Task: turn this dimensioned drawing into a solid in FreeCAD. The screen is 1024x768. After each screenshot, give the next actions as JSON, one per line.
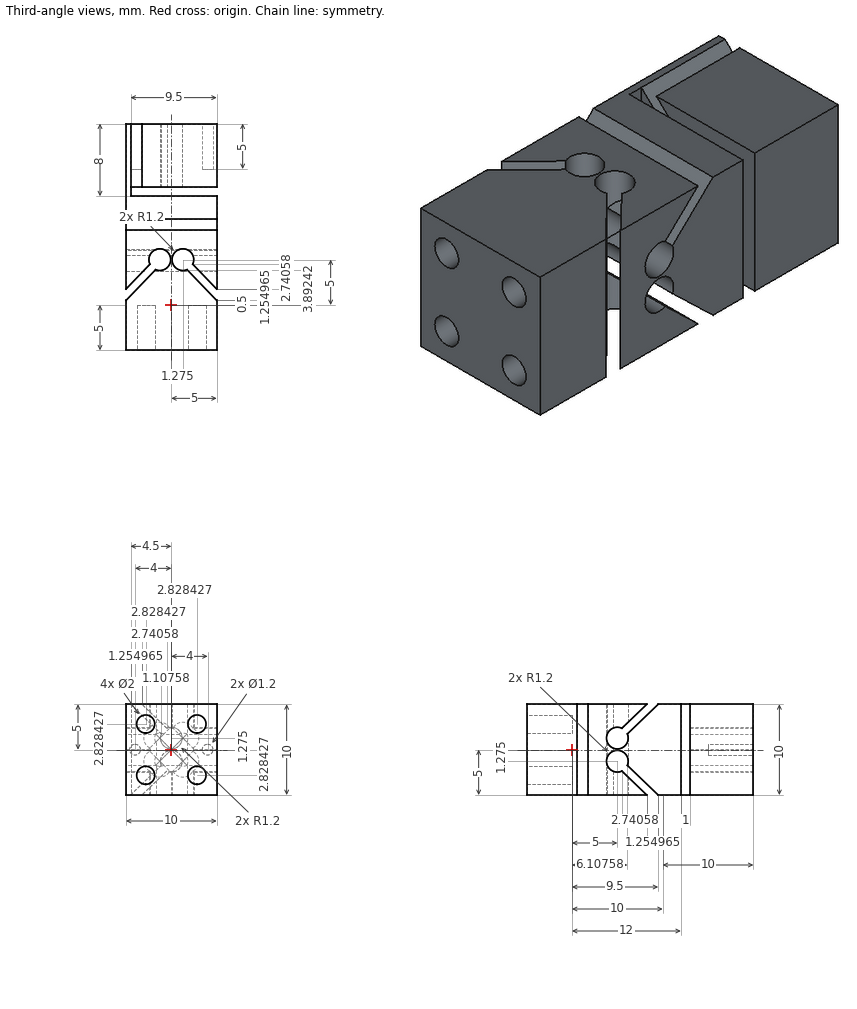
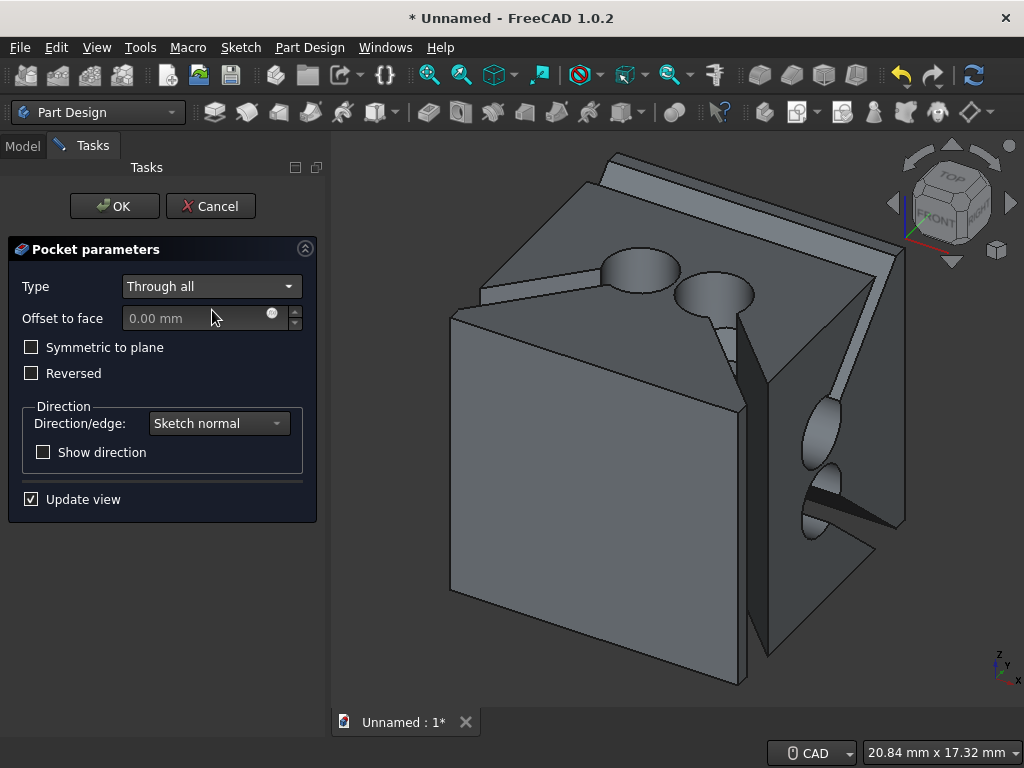
{"action": "left_click", "coordinate": [115, 206]}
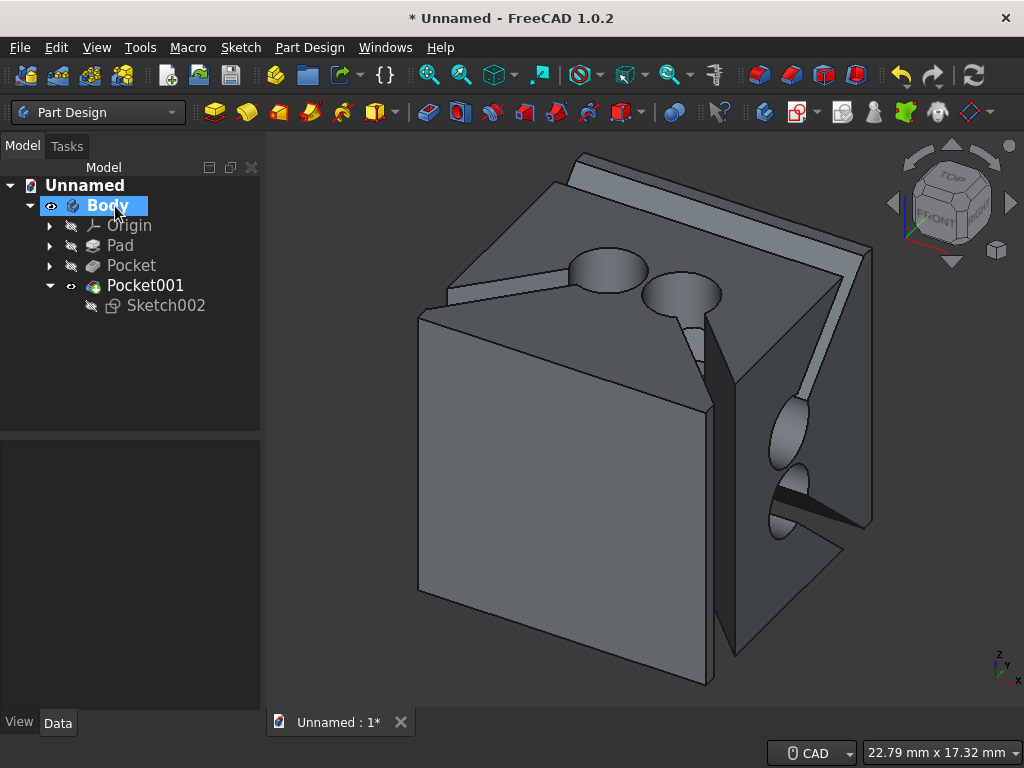
{"action": "left_click", "coordinate": [798, 112]}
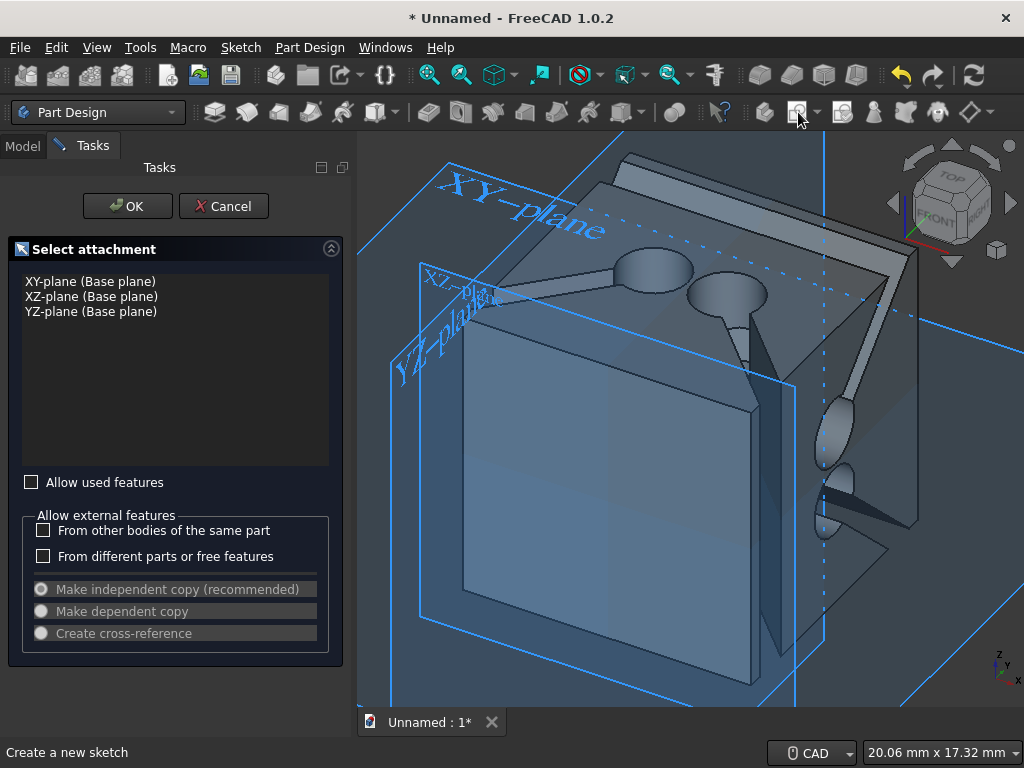
{"action": "left_click", "coordinate": [82, 296]}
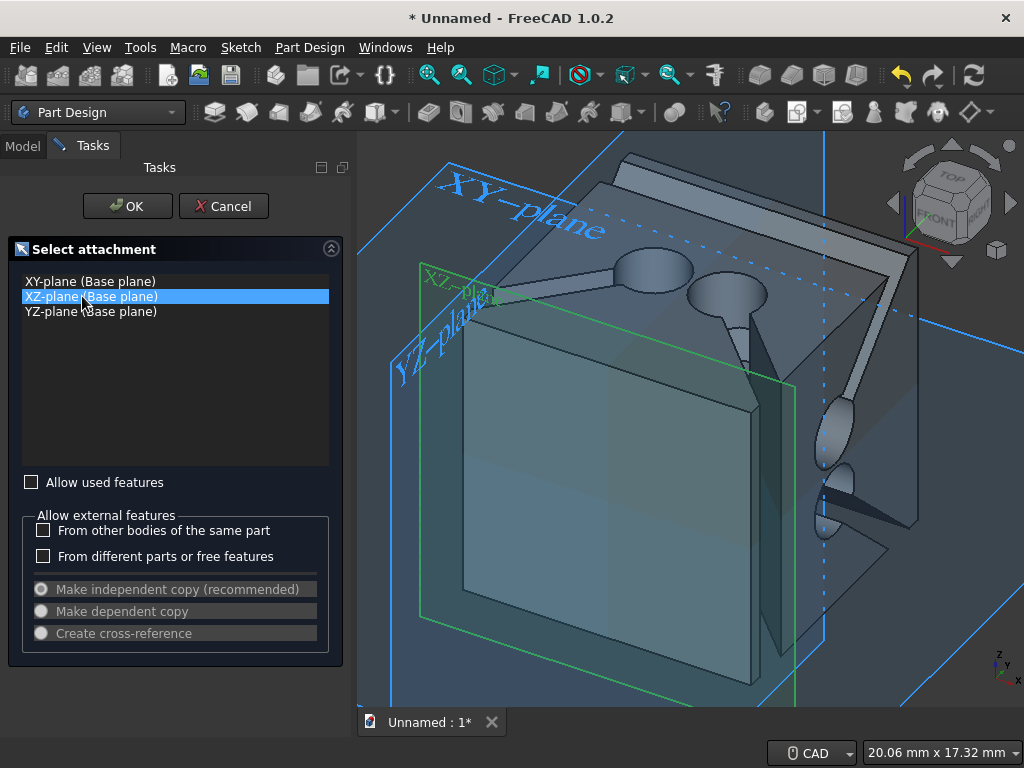
{"action": "left_click", "coordinate": [128, 206]}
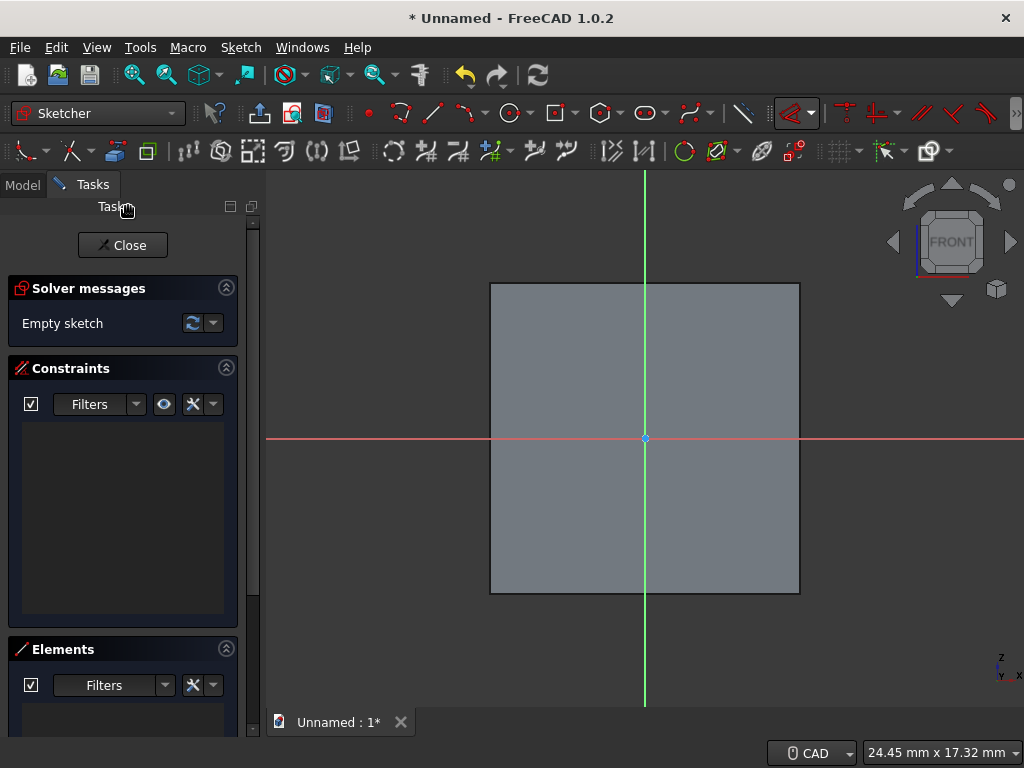
{"action": "left_click", "coordinate": [556, 114]}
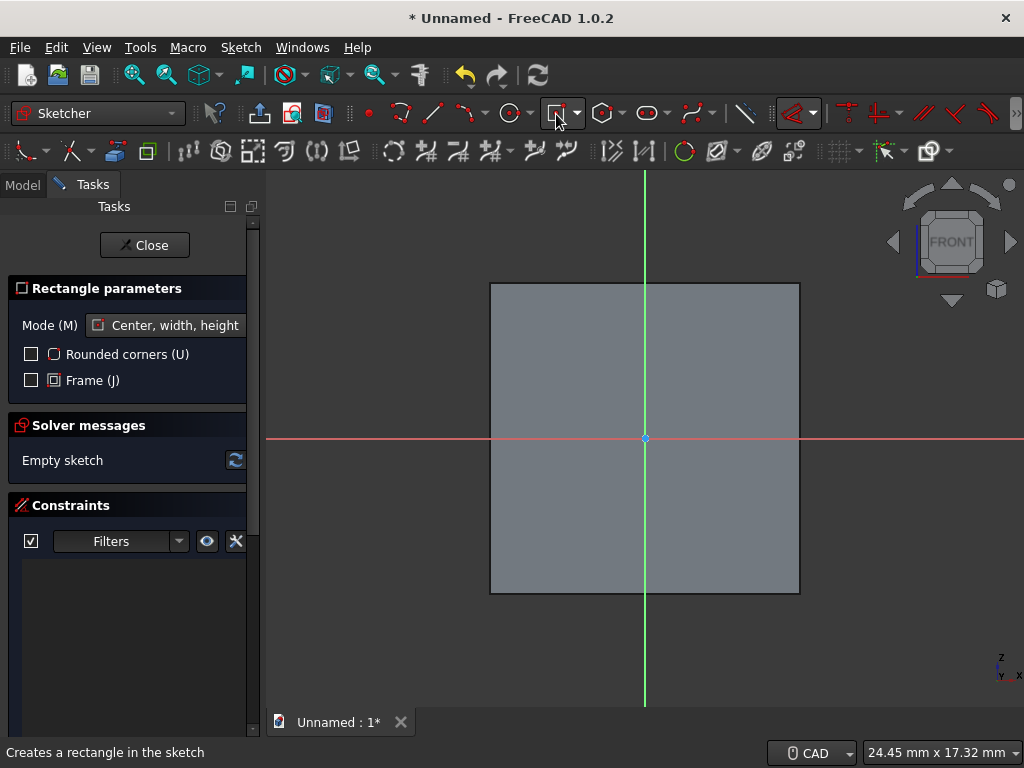
{"action": "left_click", "coordinate": [645, 439]}
{"action": "left_click", "coordinate": [800, 283]}
{"action": "key", "text": "Escape"}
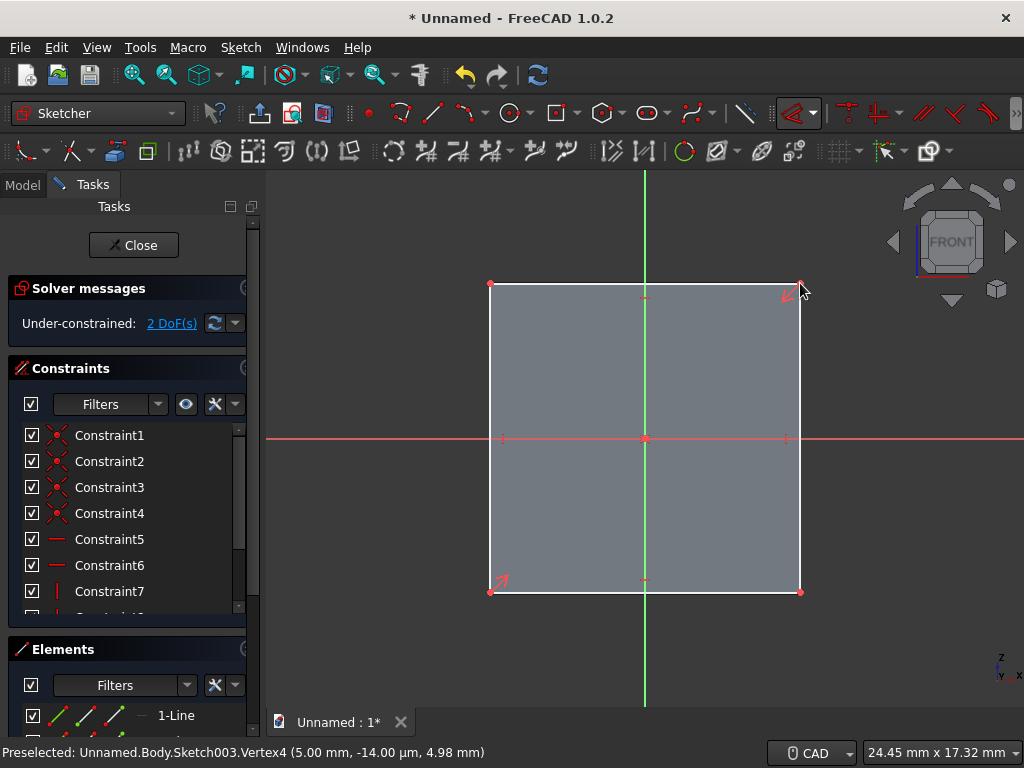
{"action": "left_click", "coordinate": [583, 593]}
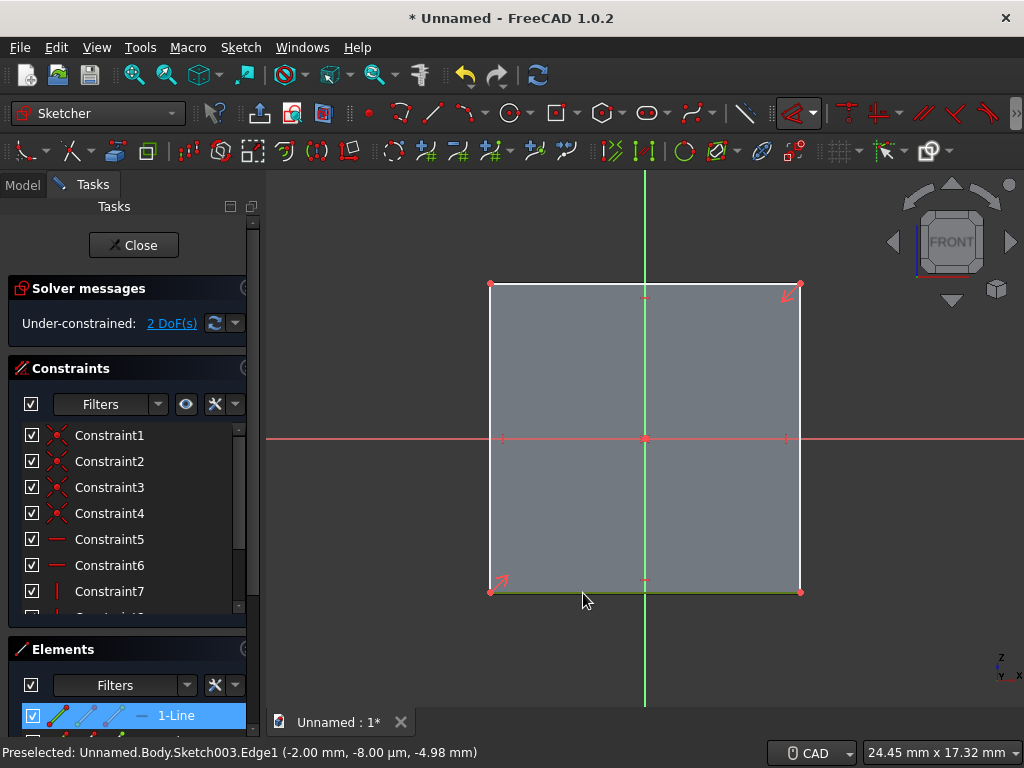
{"action": "left_click", "coordinate": [816, 114]}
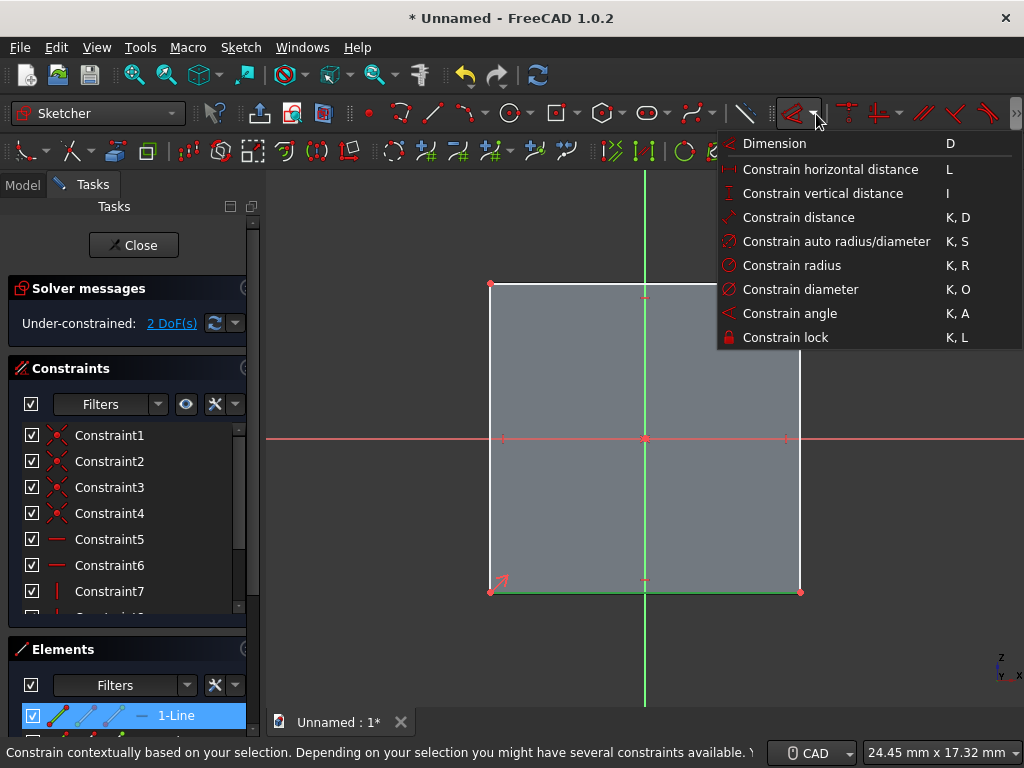
{"action": "left_click", "coordinate": [870, 169]}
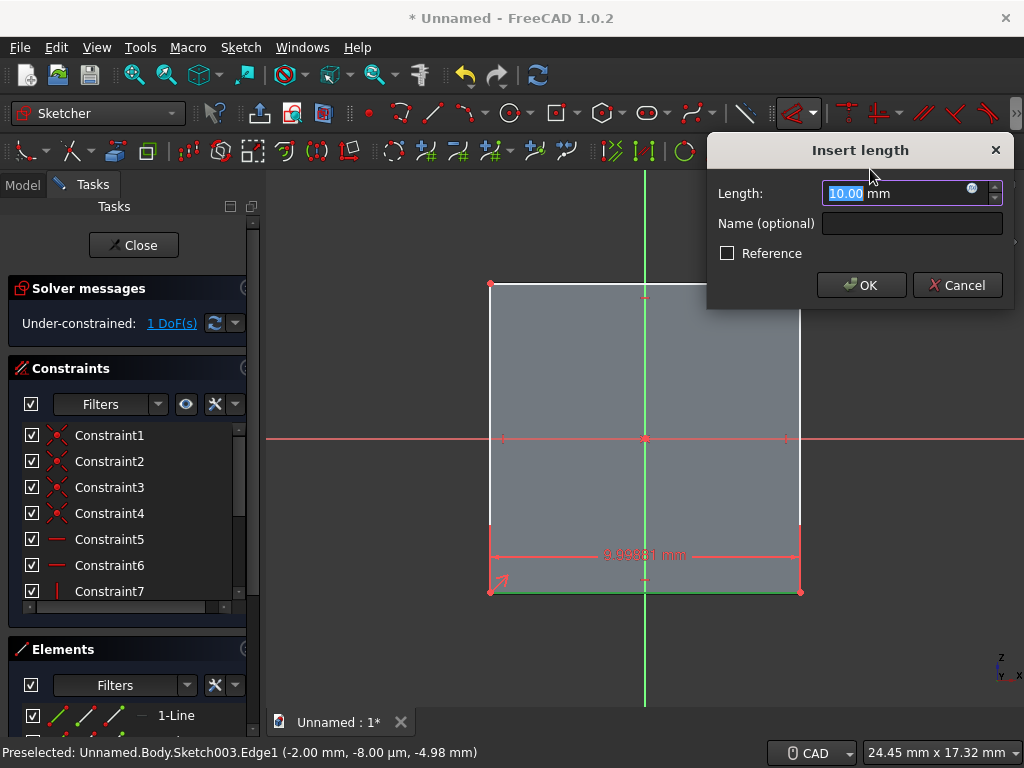
{"action": "type", "text": "10"}
{"action": "key", "text": "Return"}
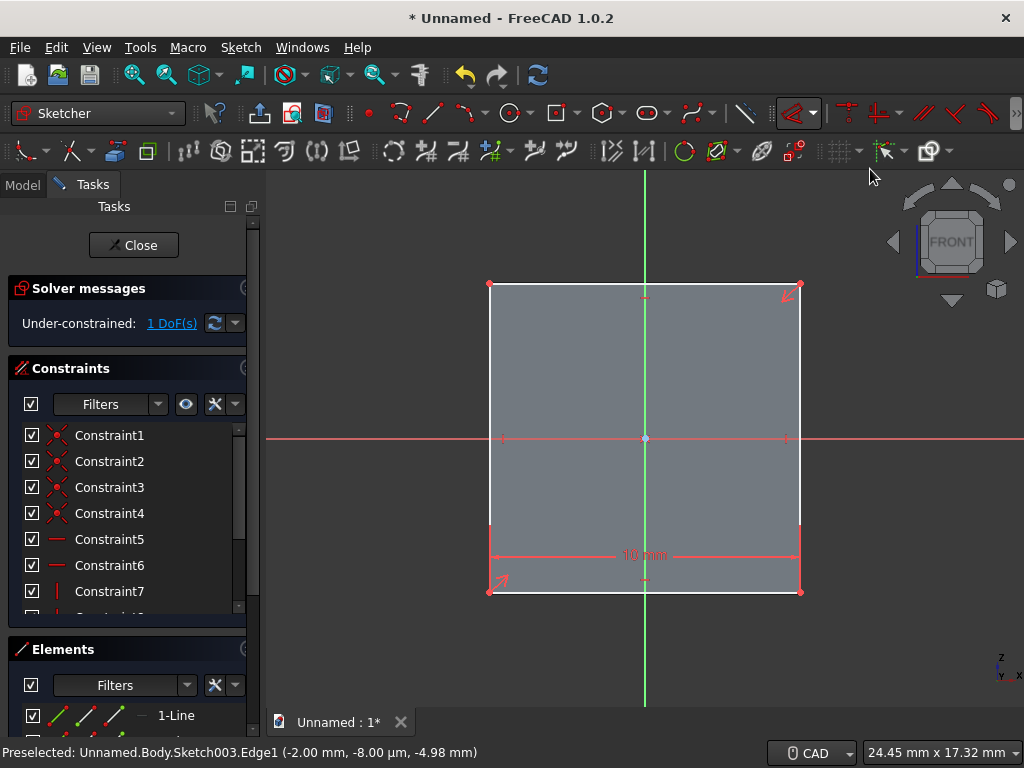
{"action": "left_click", "coordinate": [800, 500]}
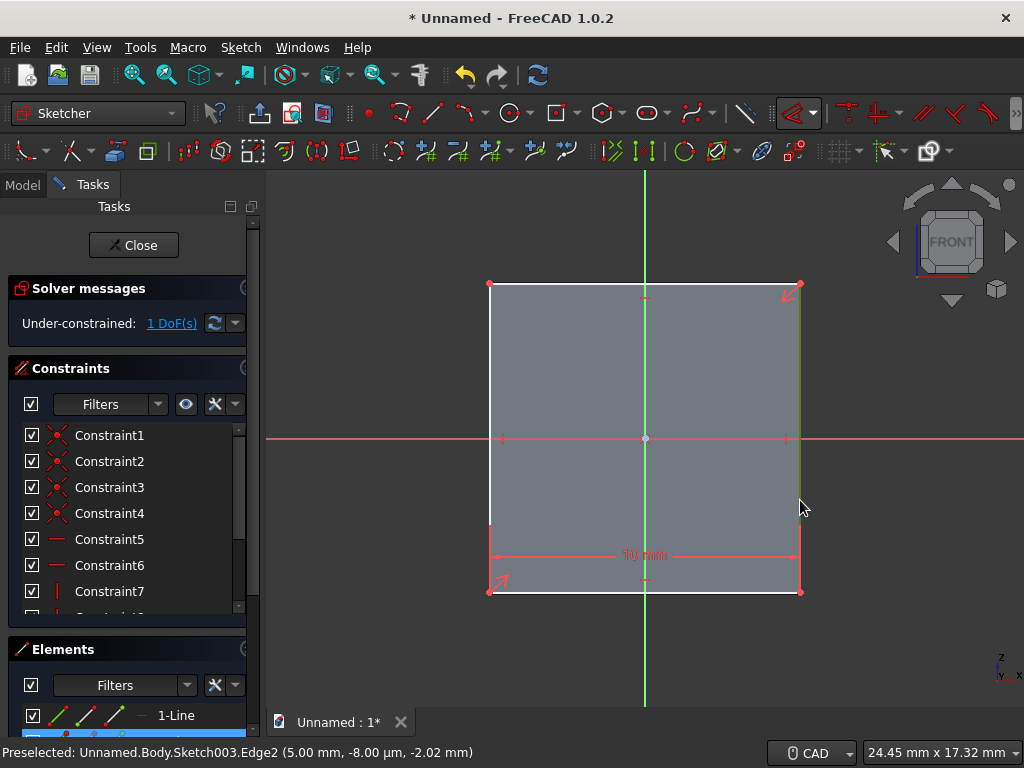
{"action": "key", "text": "i"}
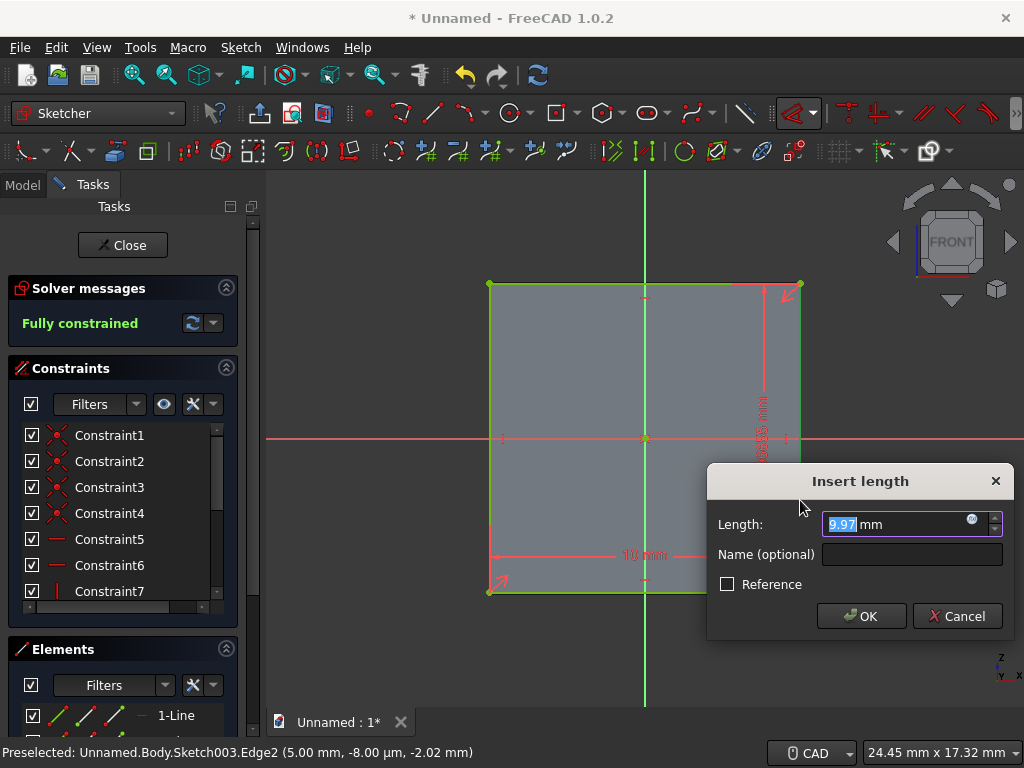
{"action": "type", "text": "10"}
{"action": "key", "text": "Return"}